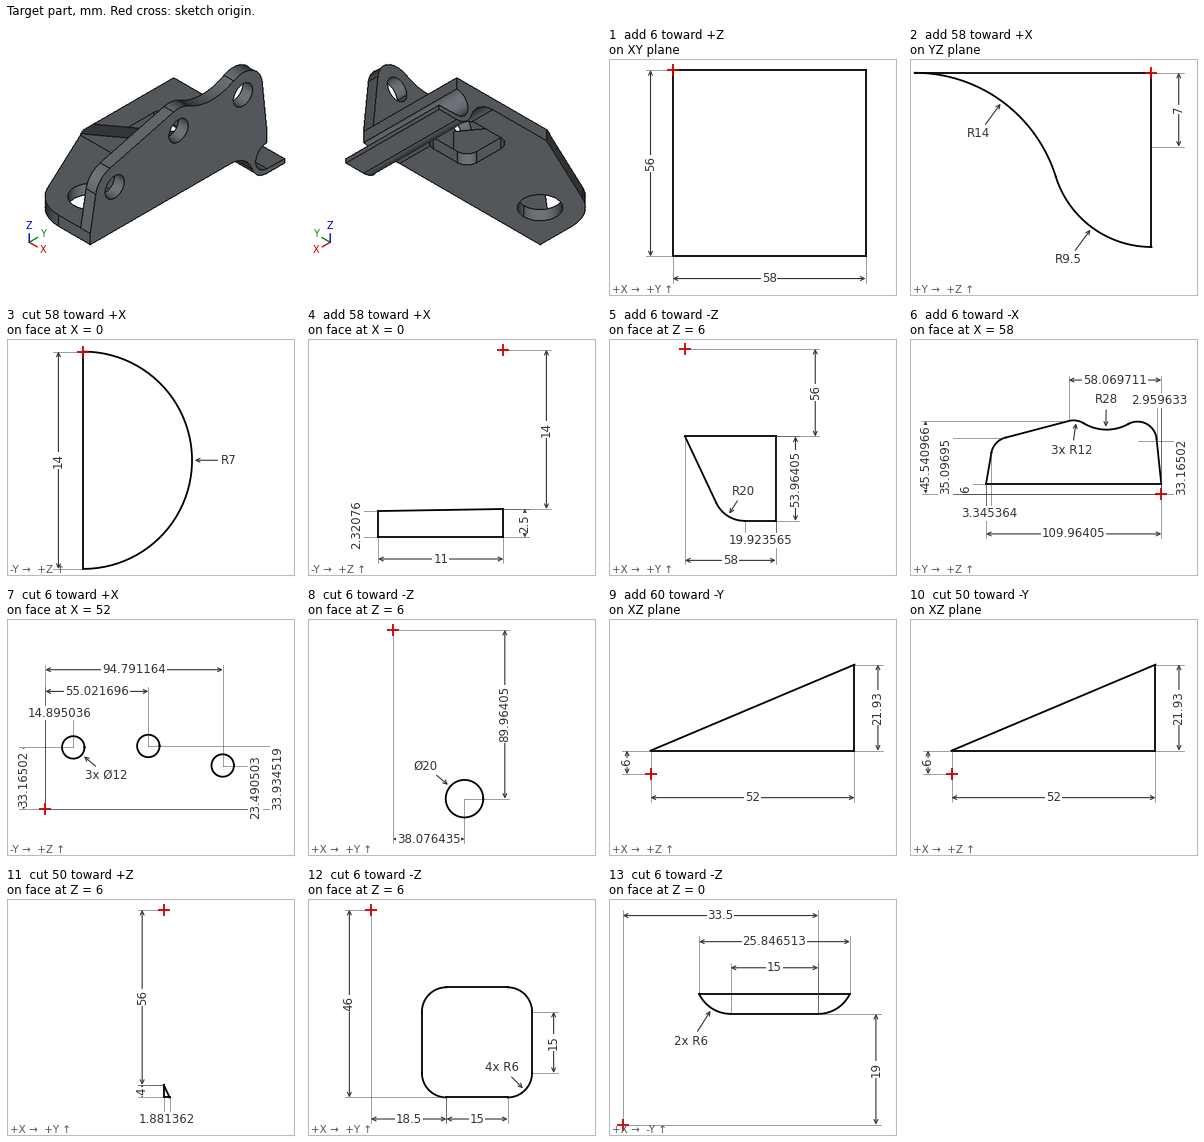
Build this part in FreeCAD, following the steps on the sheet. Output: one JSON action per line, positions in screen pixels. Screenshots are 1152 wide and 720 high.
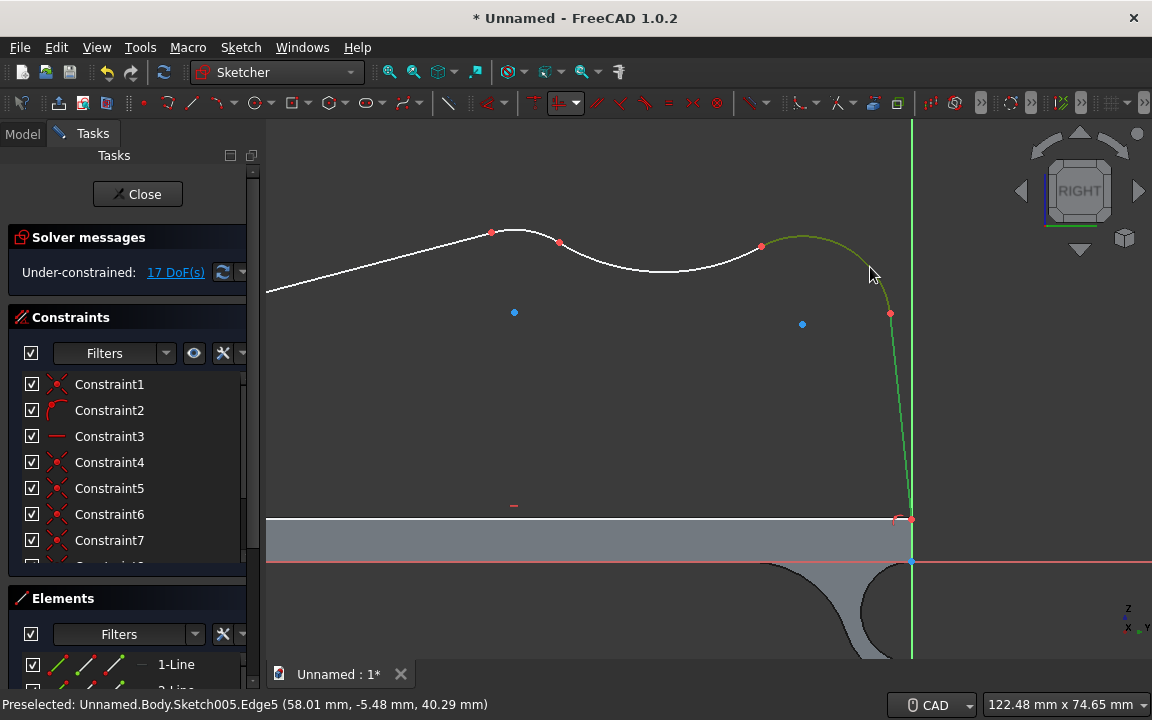
{"action": "left_click", "coordinate": [646, 104]}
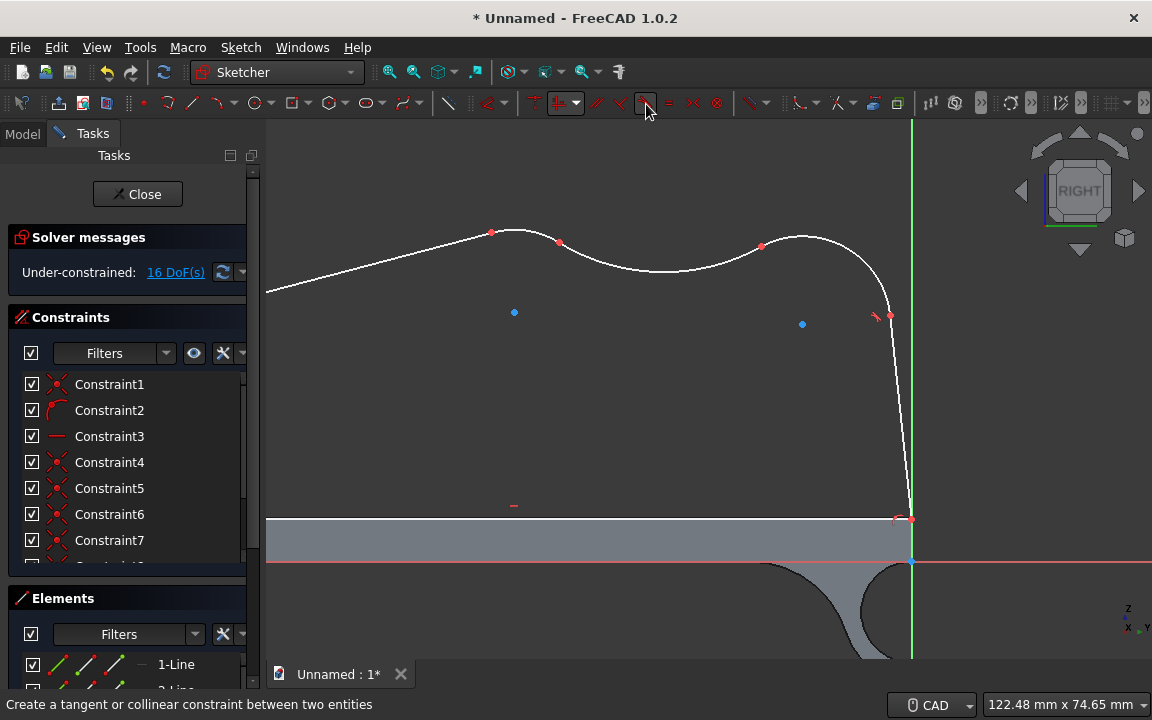
{"action": "left_click", "coordinate": [405, 256]}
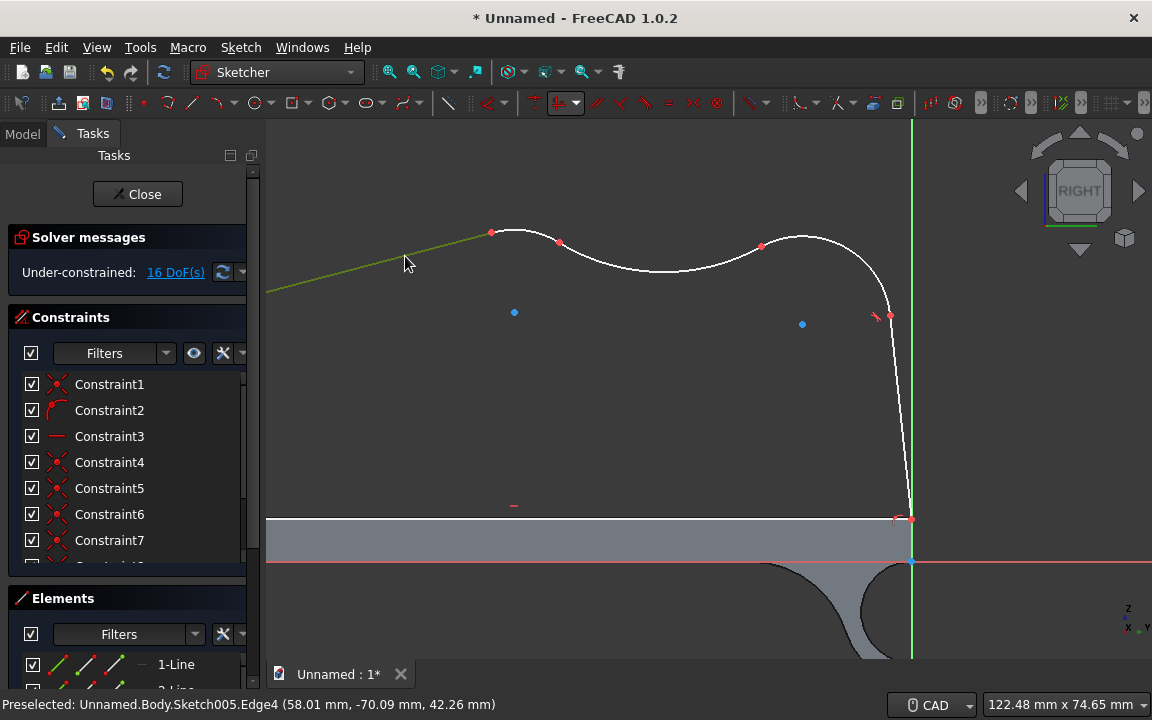
{"action": "left_click", "coordinate": [540, 234]}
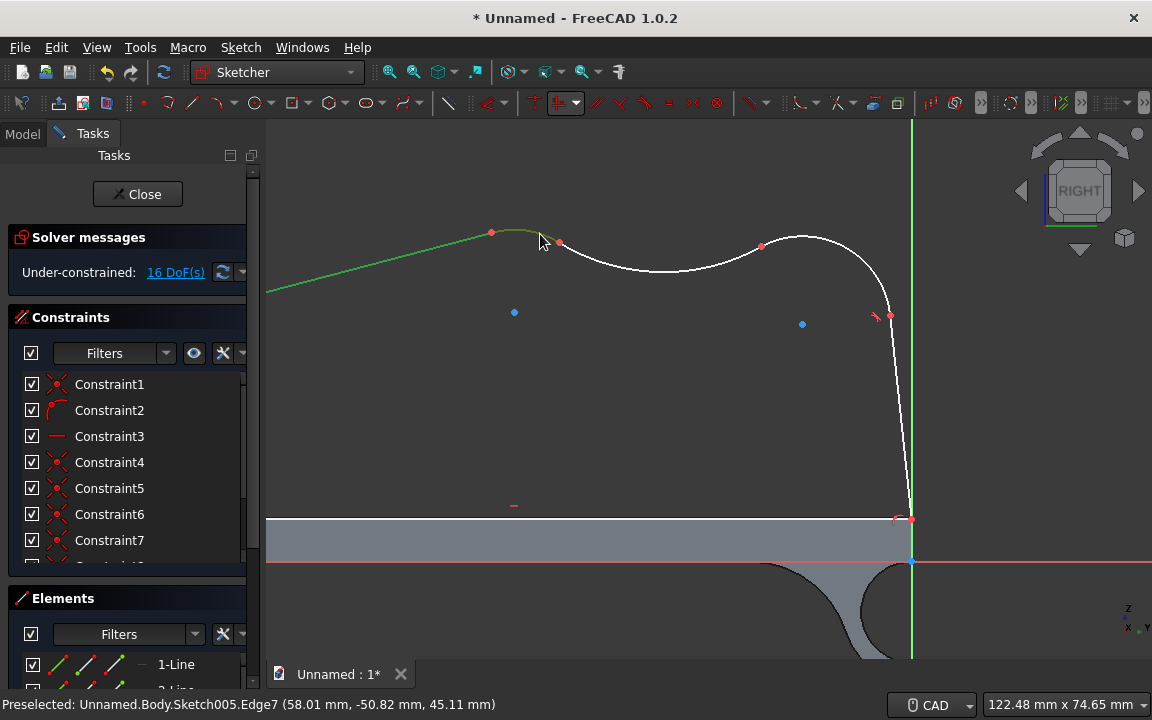
{"action": "left_click", "coordinate": [646, 104]}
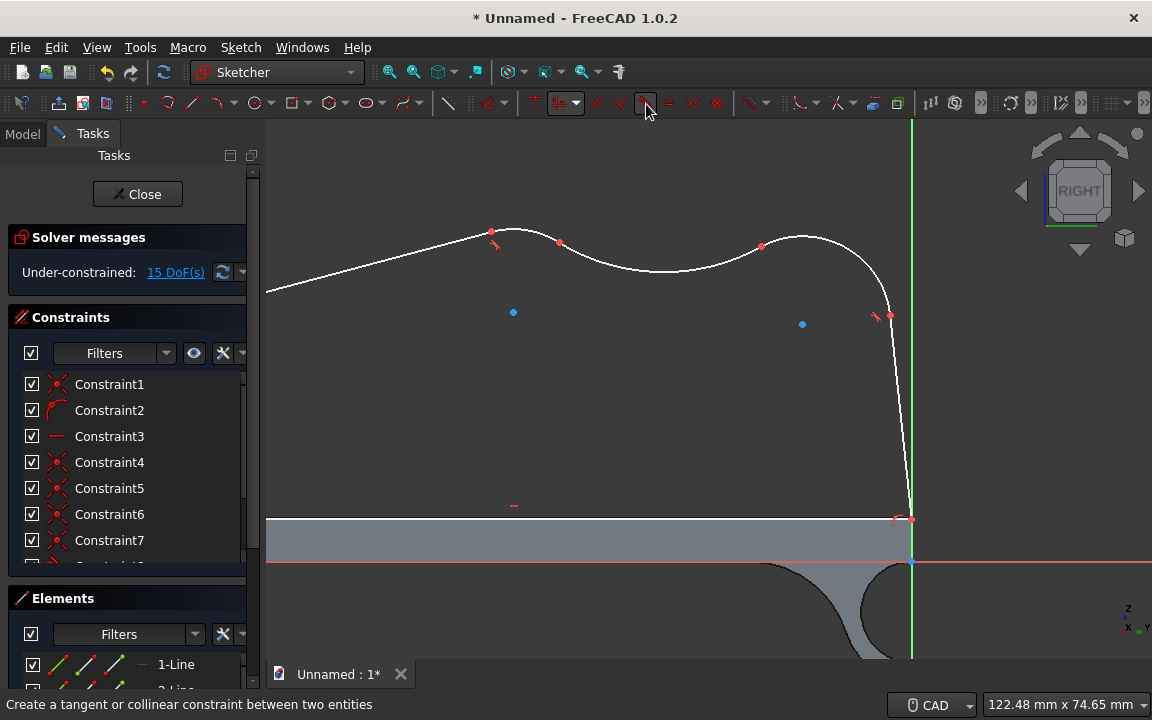
{"action": "left_click", "coordinate": [405, 255]}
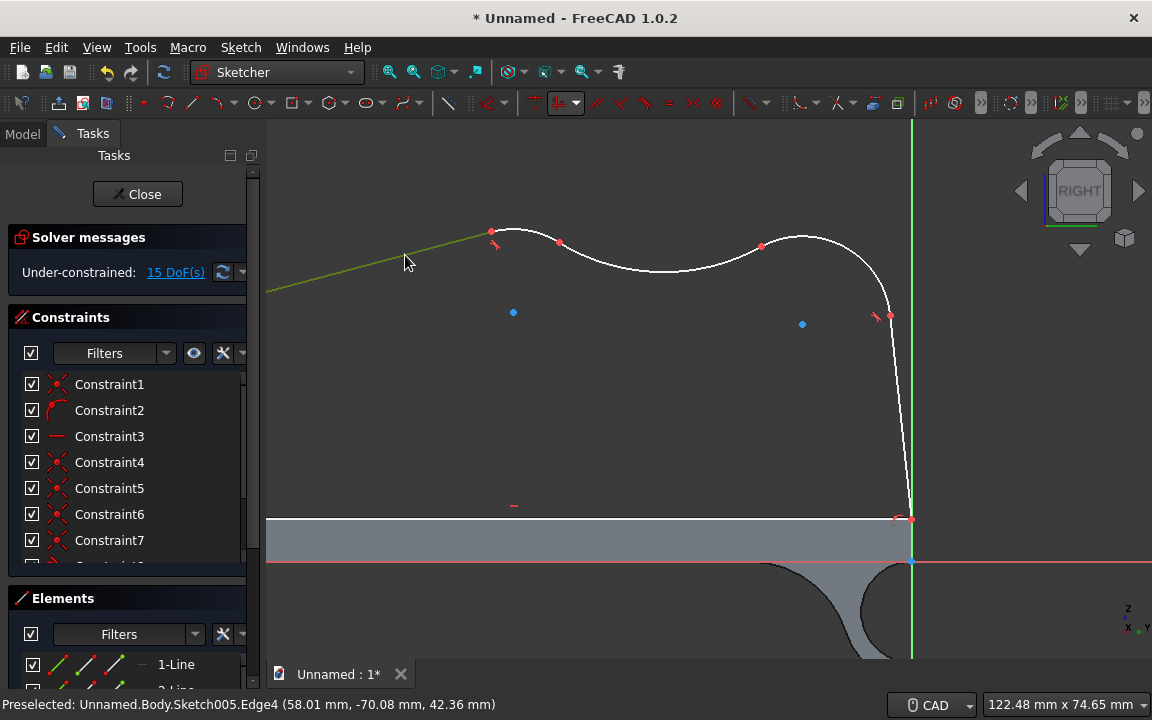
{"action": "scroll", "coordinate": [898, 375], "scroll_direction": "down", "scroll_amount": 2}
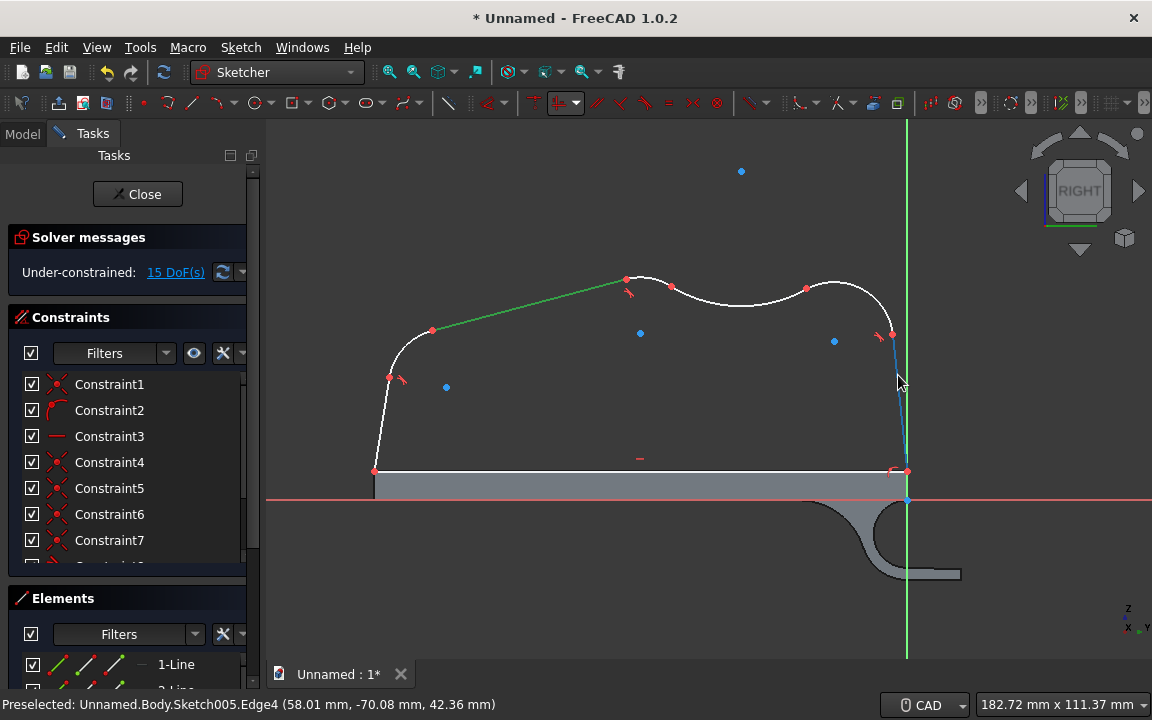
{"action": "left_click", "coordinate": [414, 339]}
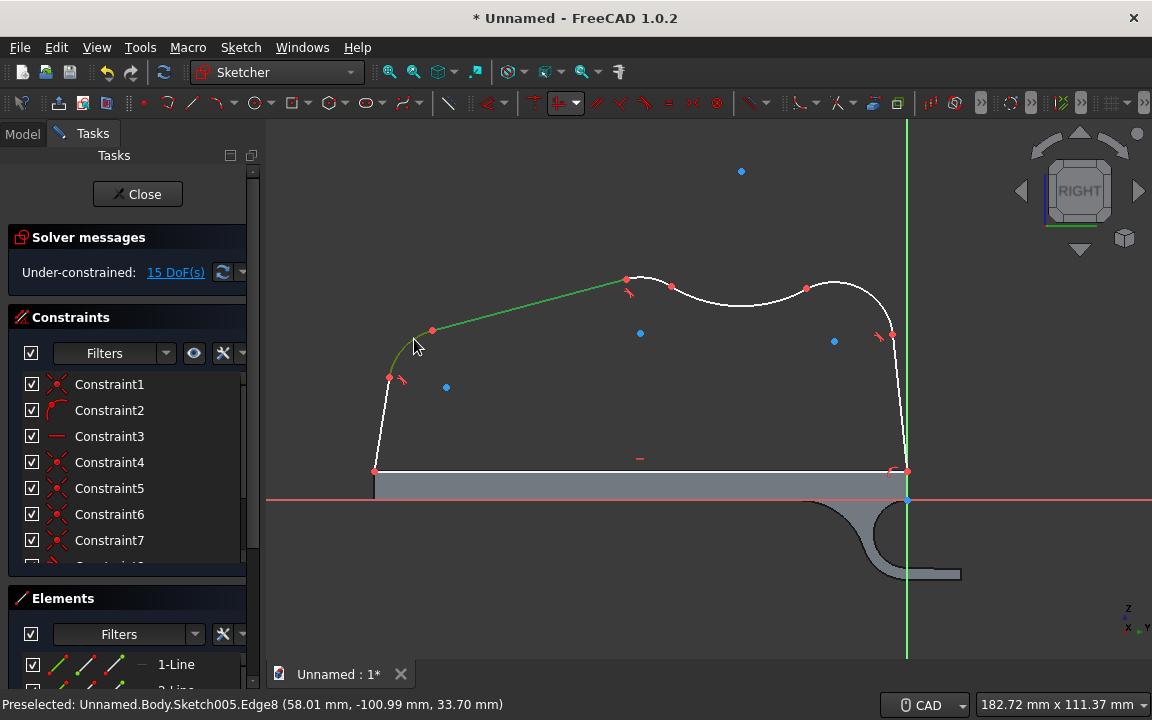
{"action": "key", "text": "t"}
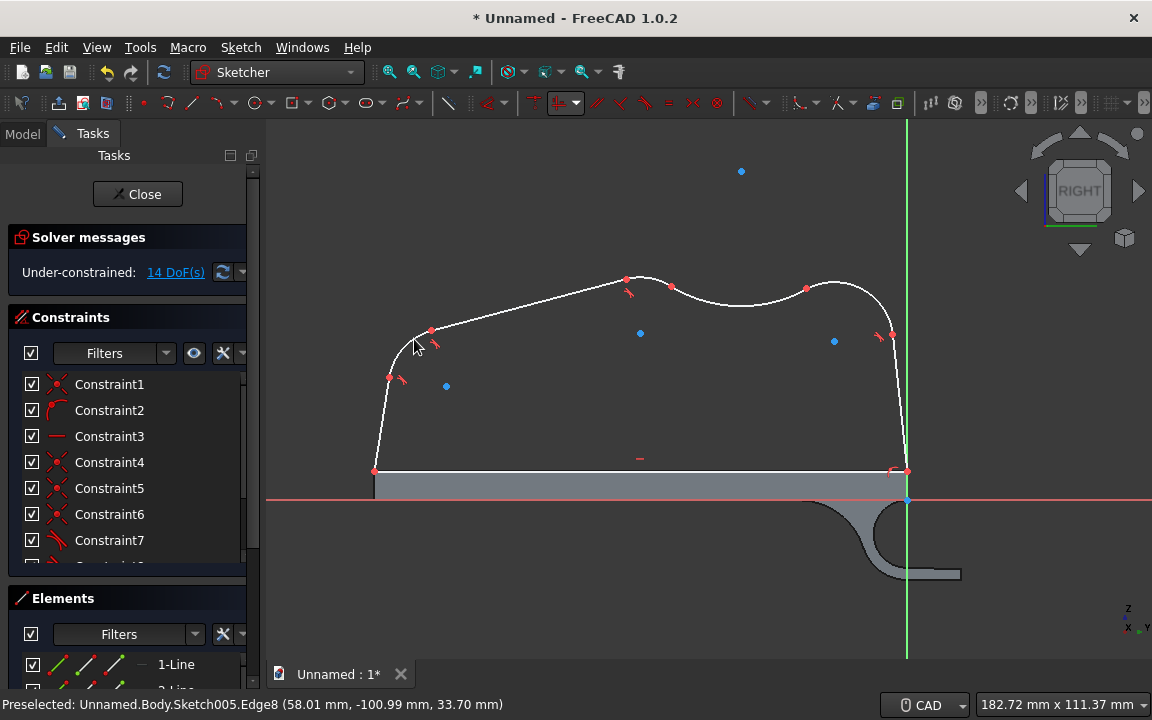
{"action": "left_click", "coordinate": [880, 304]}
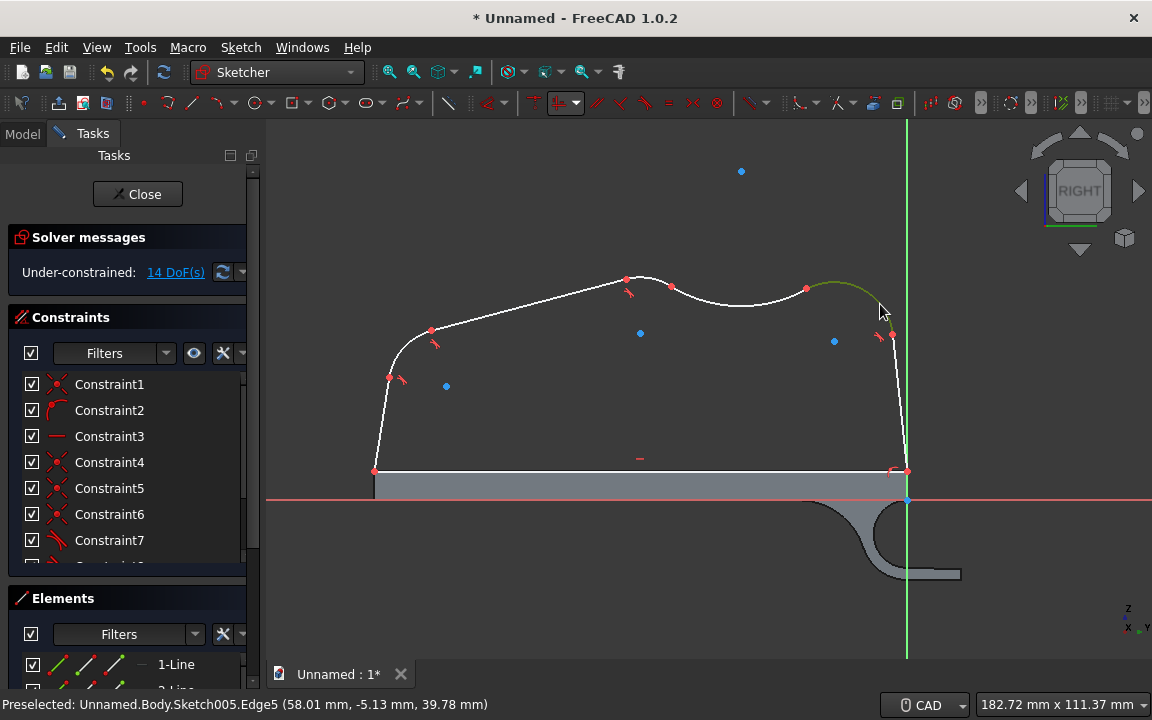
{"action": "left_click", "coordinate": [710, 303]}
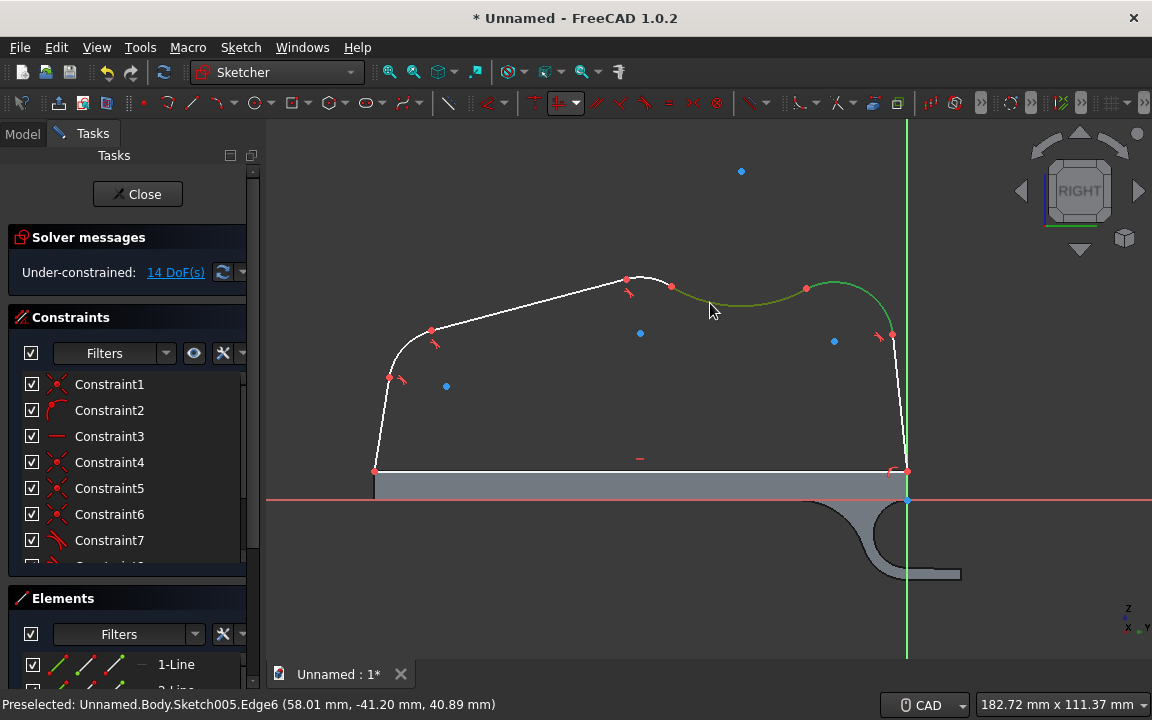
{"action": "left_click", "coordinate": [646, 104]}